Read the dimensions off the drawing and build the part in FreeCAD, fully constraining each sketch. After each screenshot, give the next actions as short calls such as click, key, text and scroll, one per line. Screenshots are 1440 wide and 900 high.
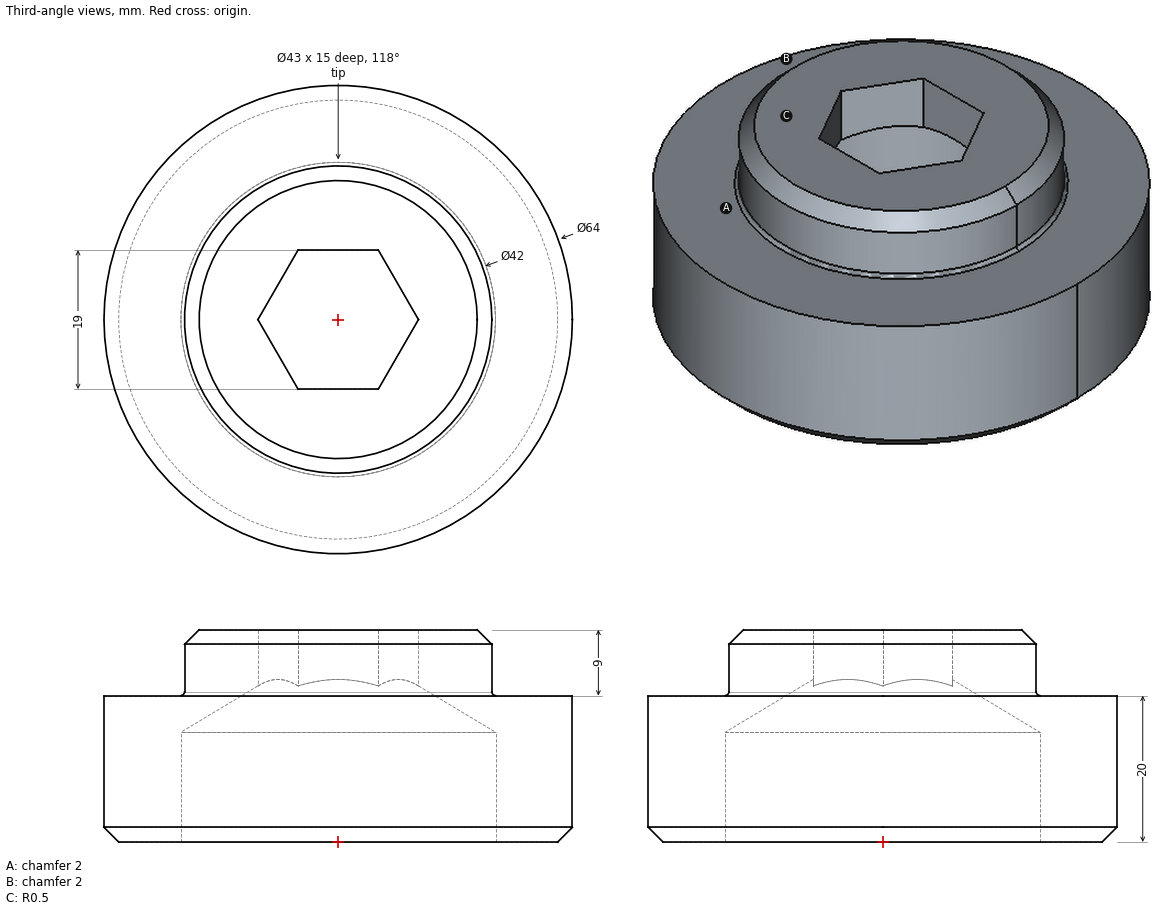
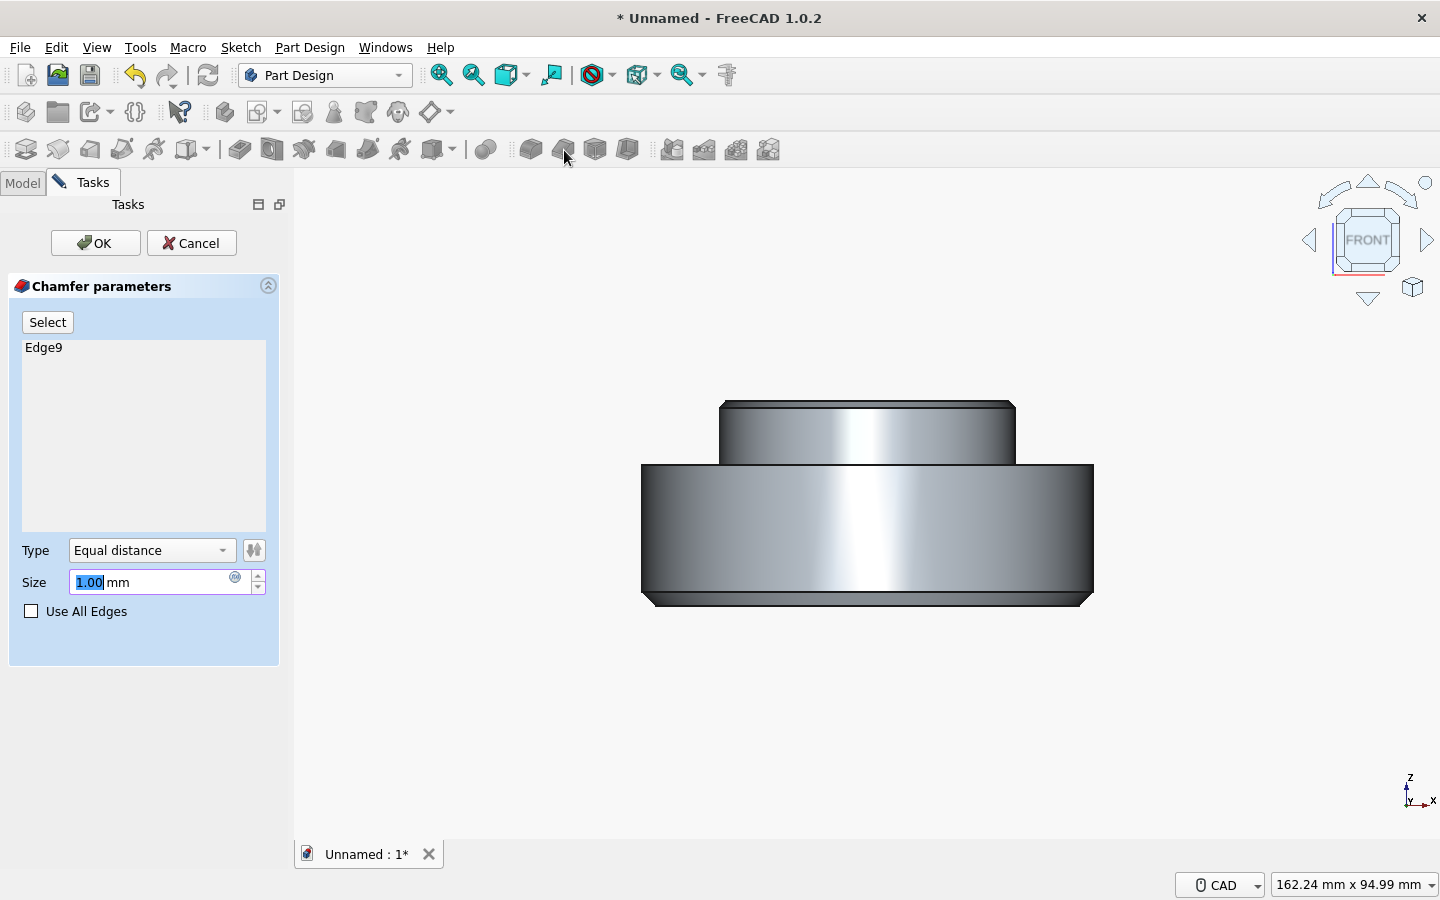
text(2)
key(Tab)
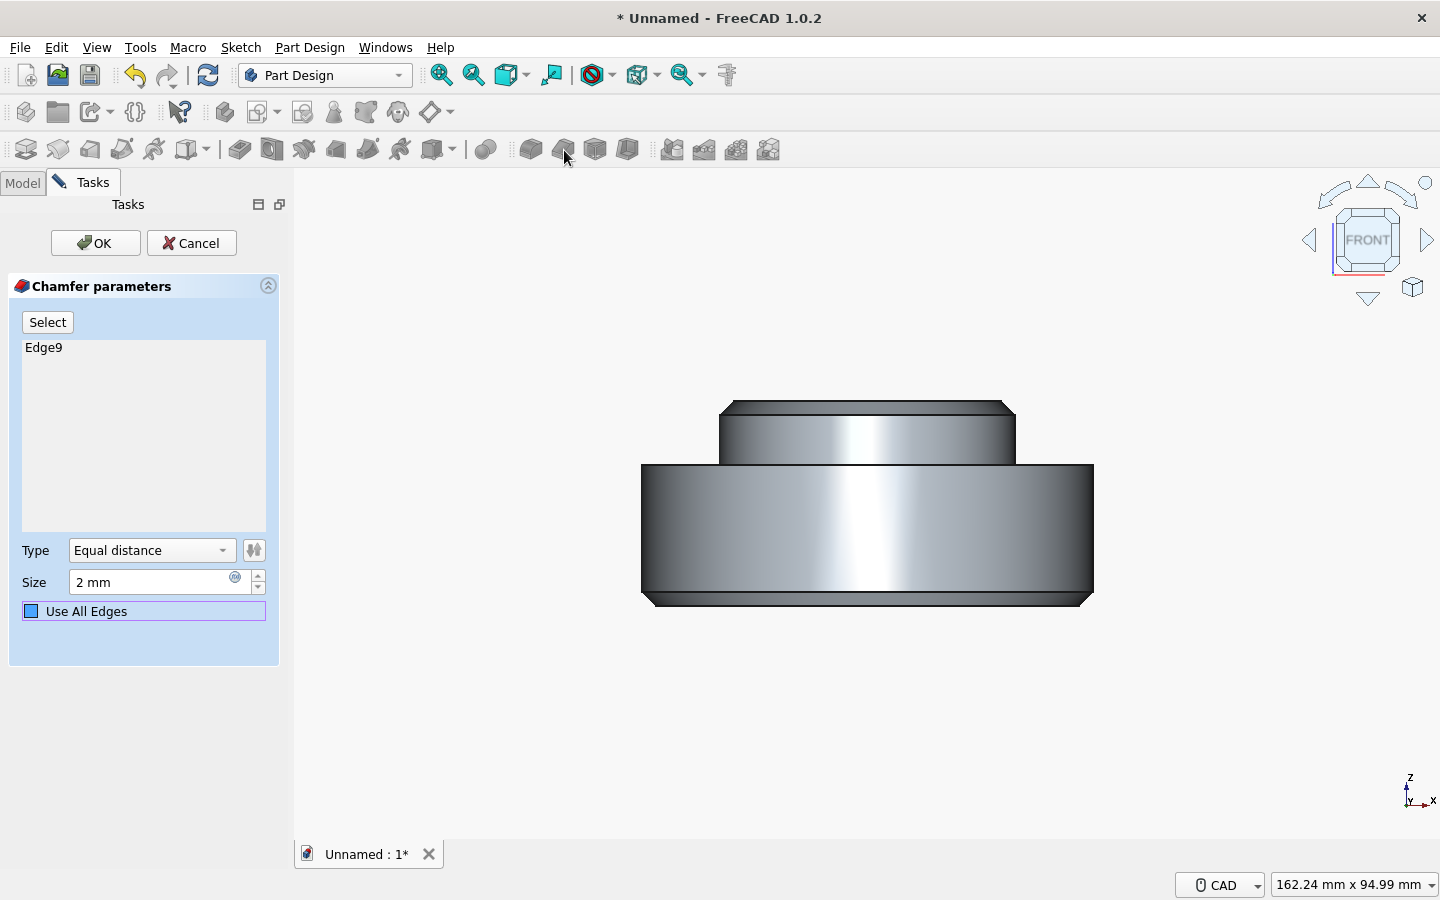
click(96, 243)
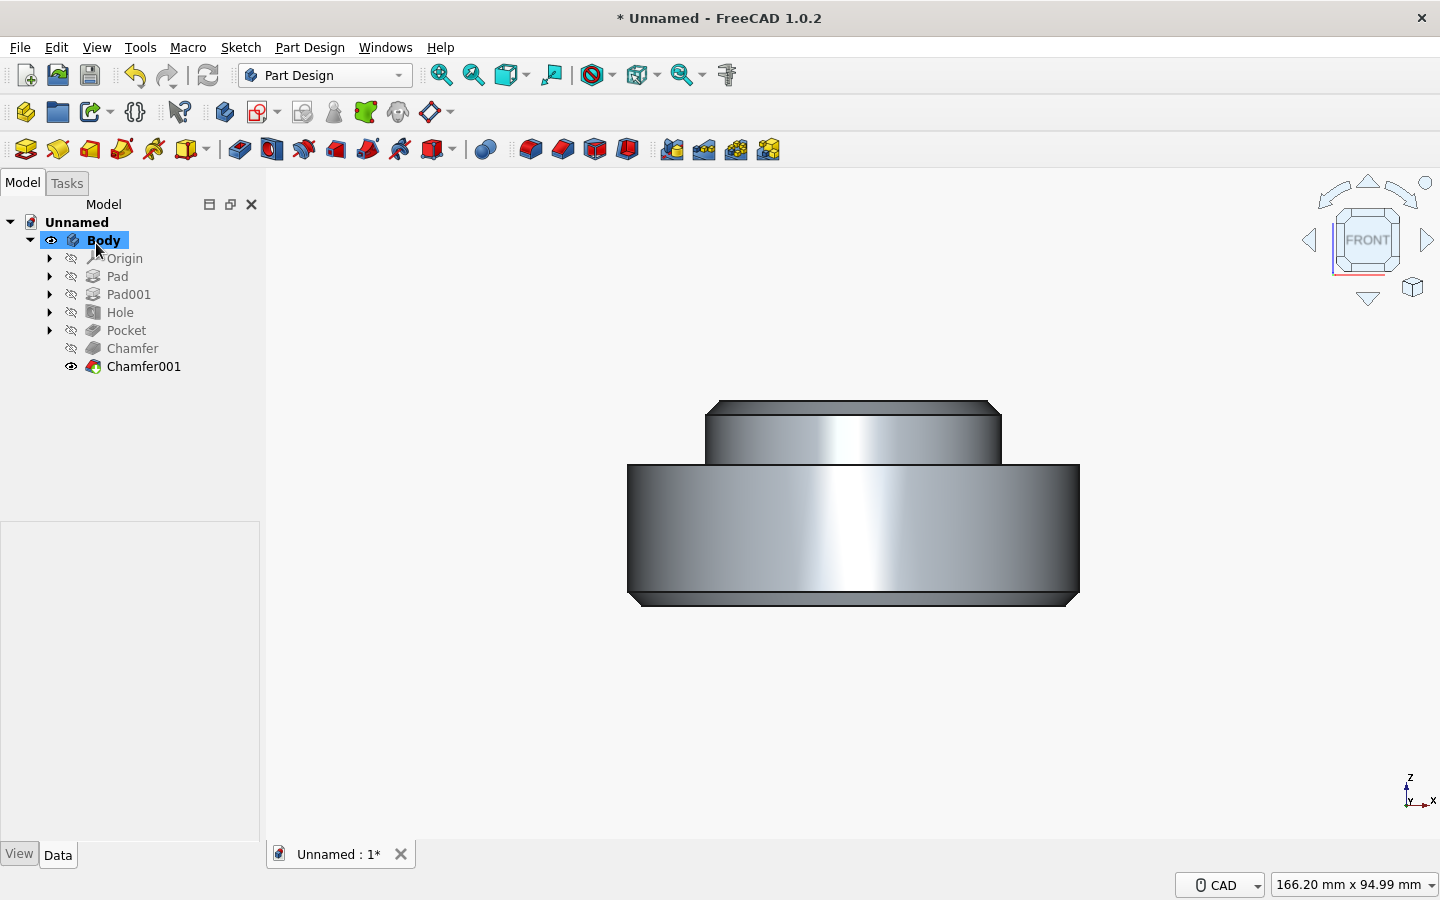
click(442, 76)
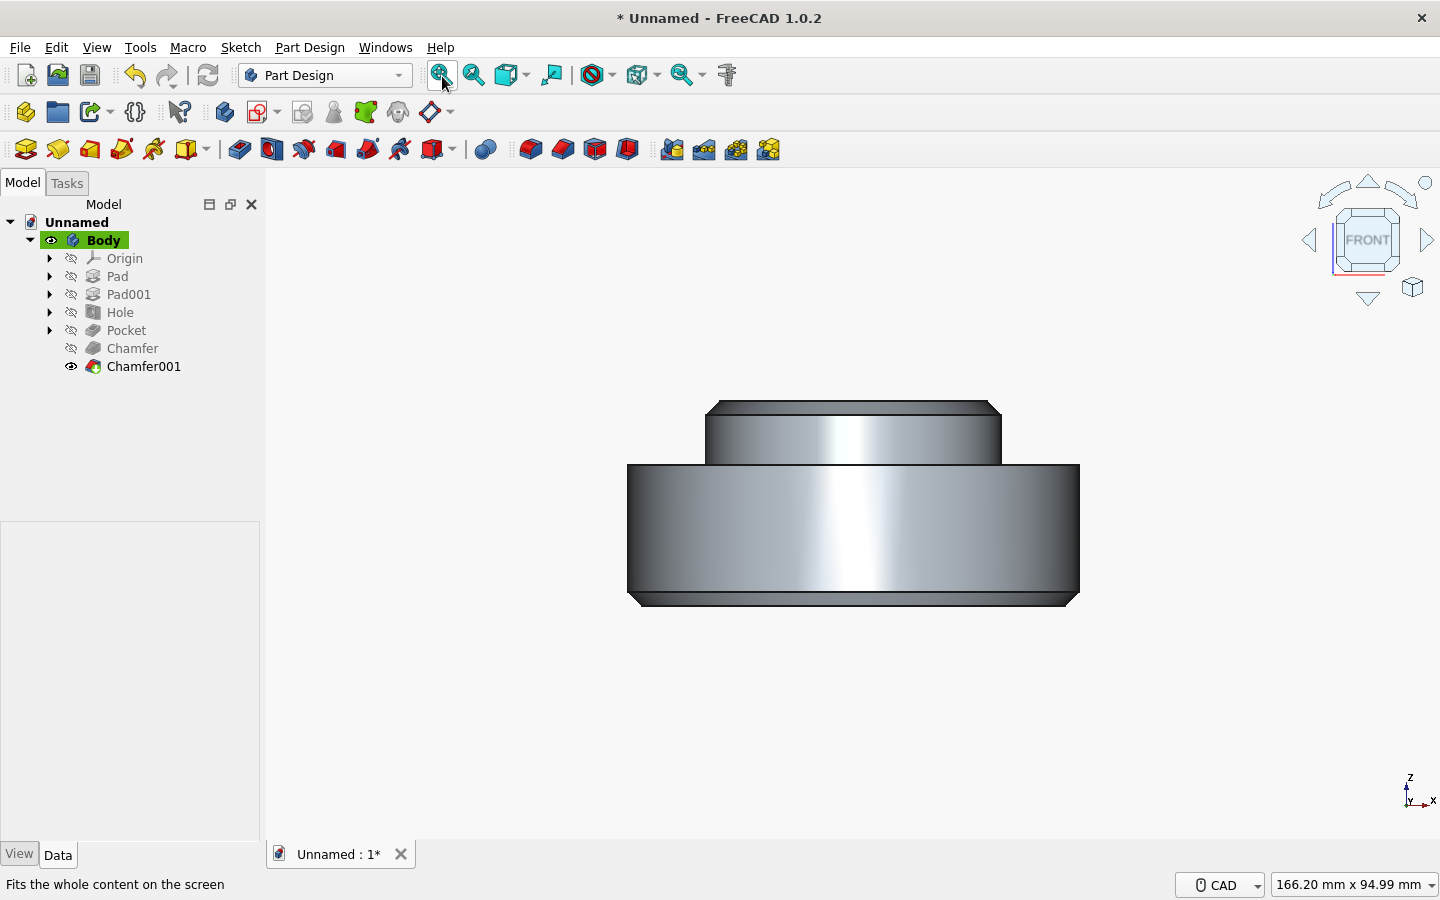
key(0)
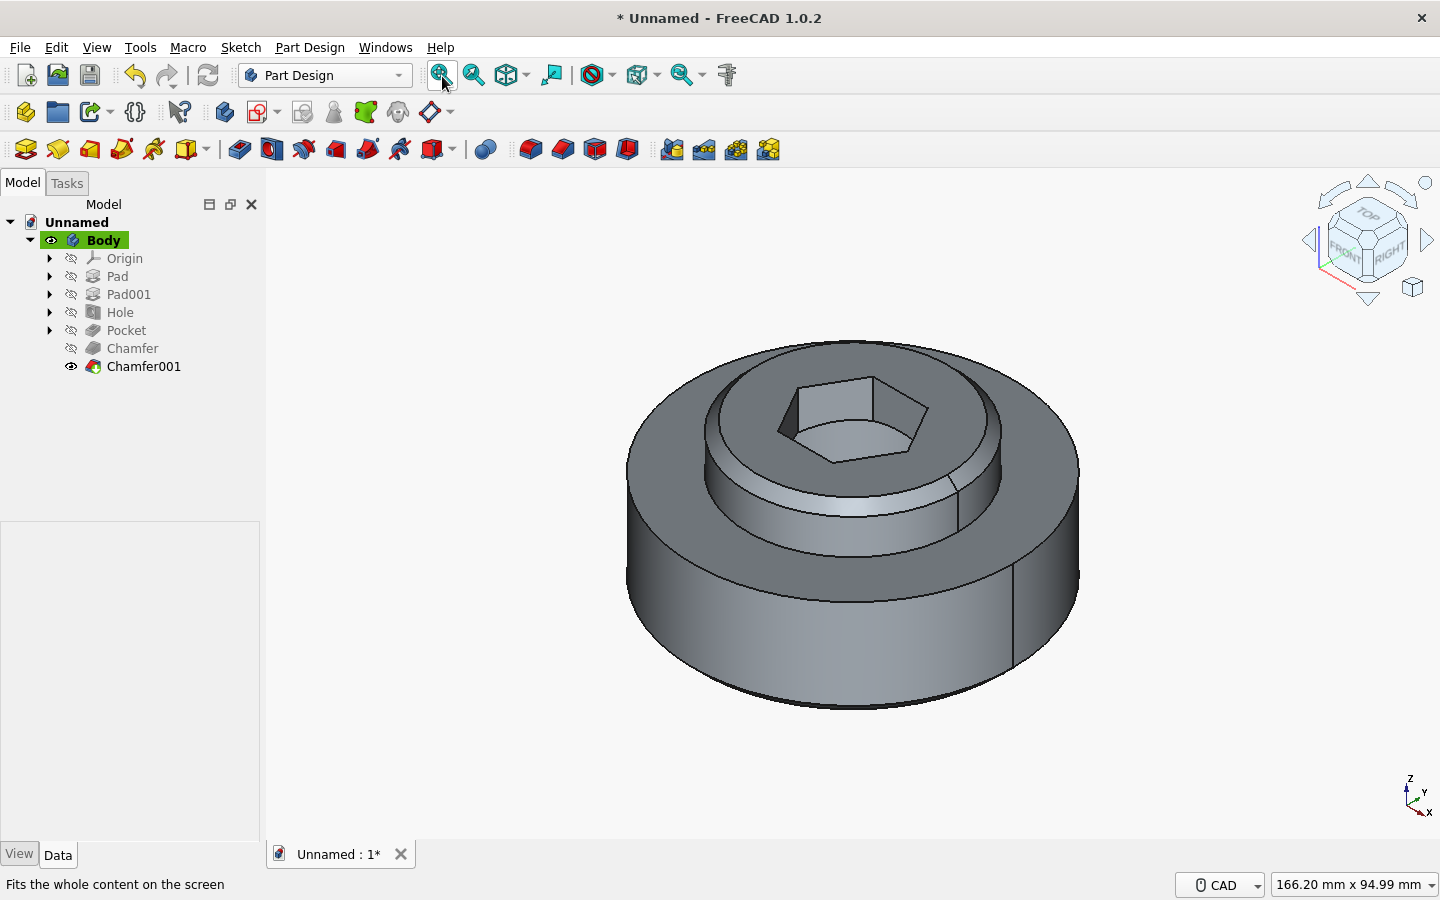
key(2)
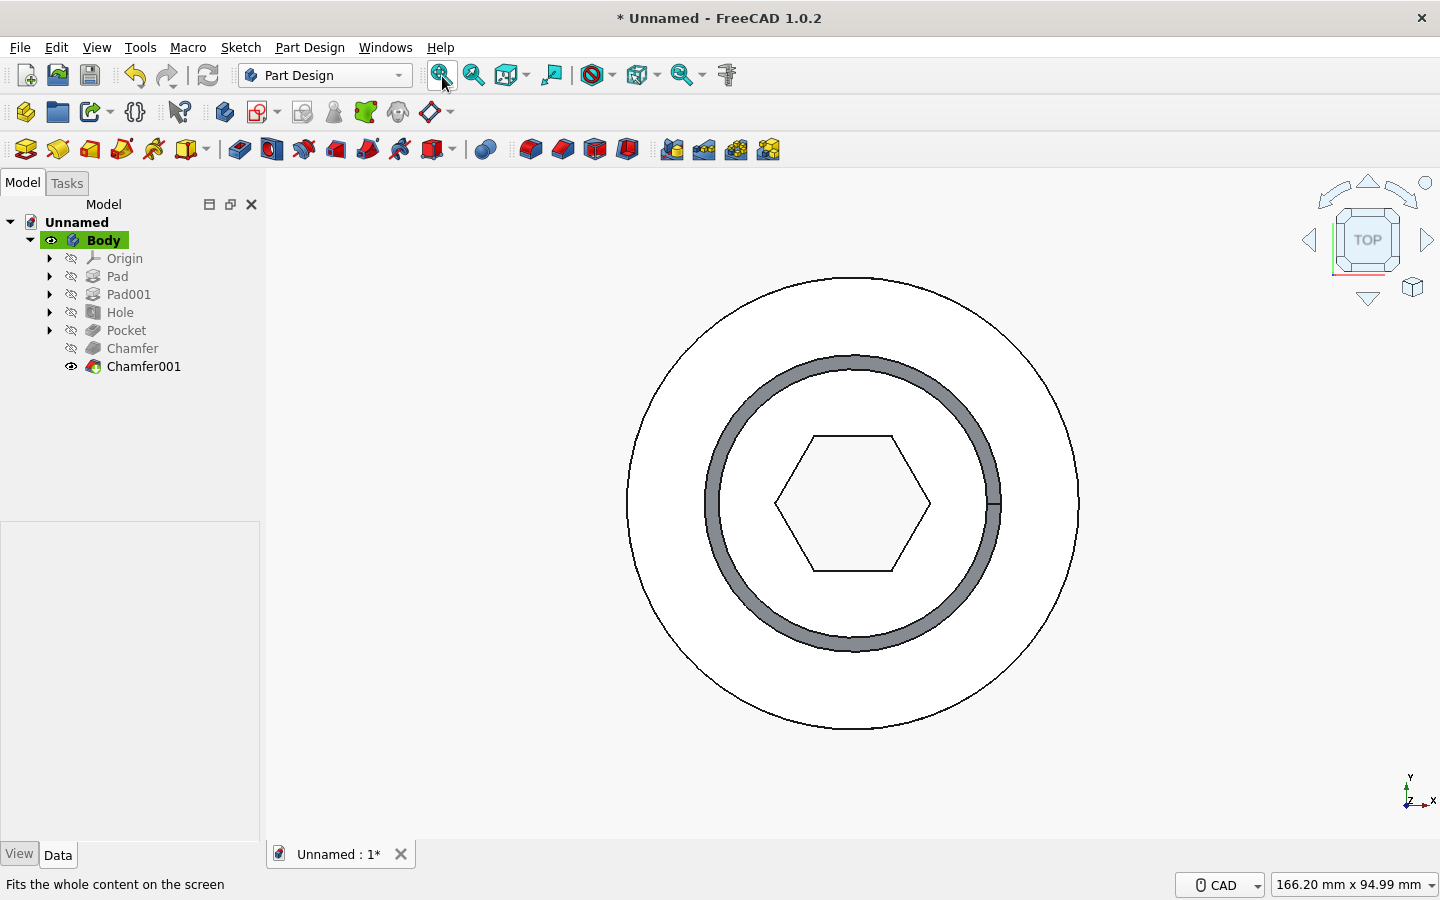
key(1)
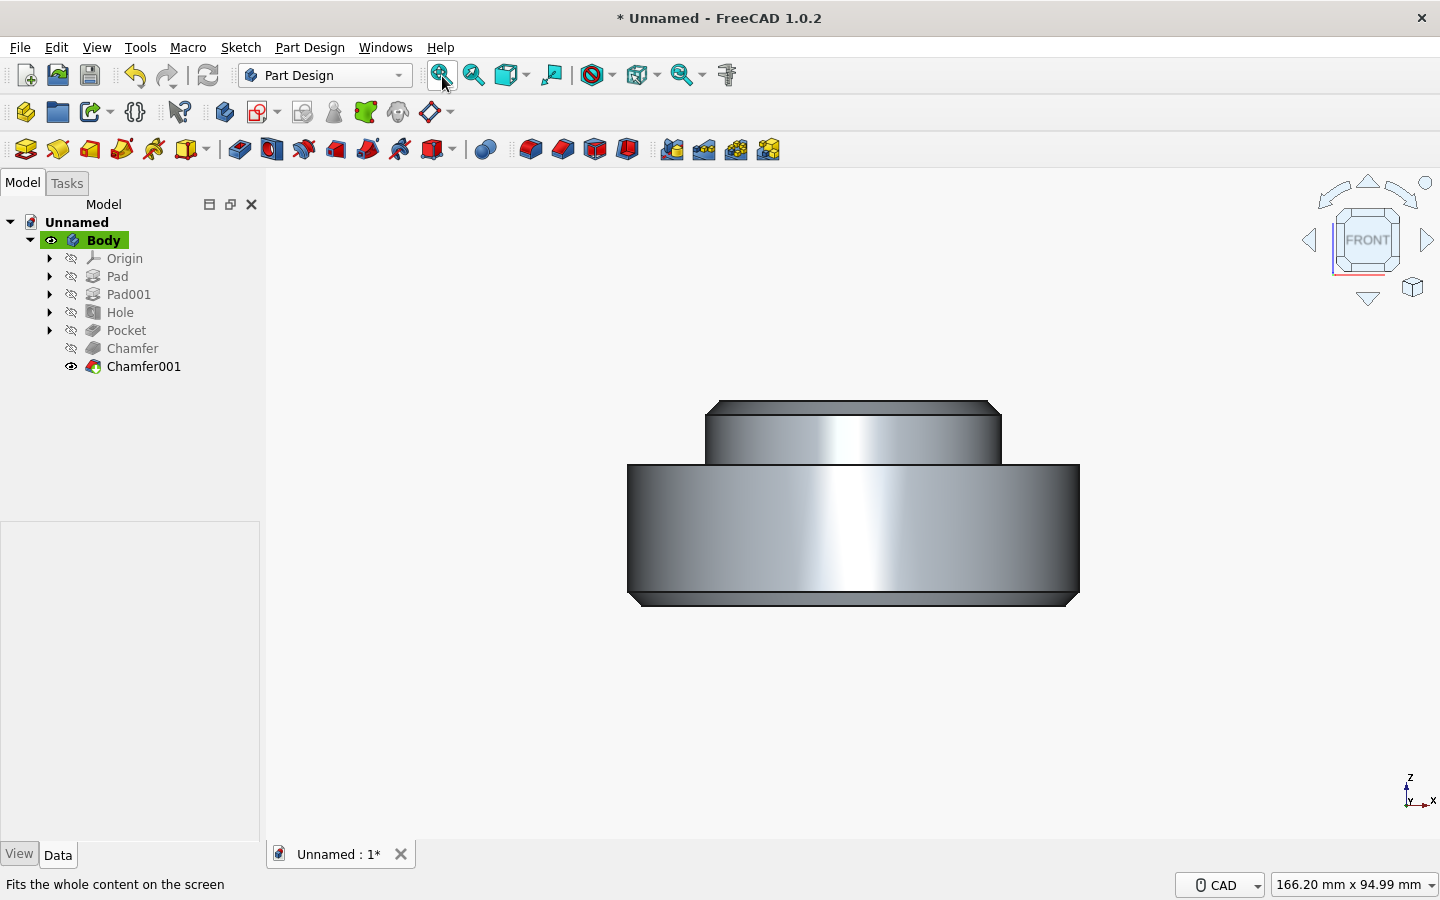
click(442, 76)